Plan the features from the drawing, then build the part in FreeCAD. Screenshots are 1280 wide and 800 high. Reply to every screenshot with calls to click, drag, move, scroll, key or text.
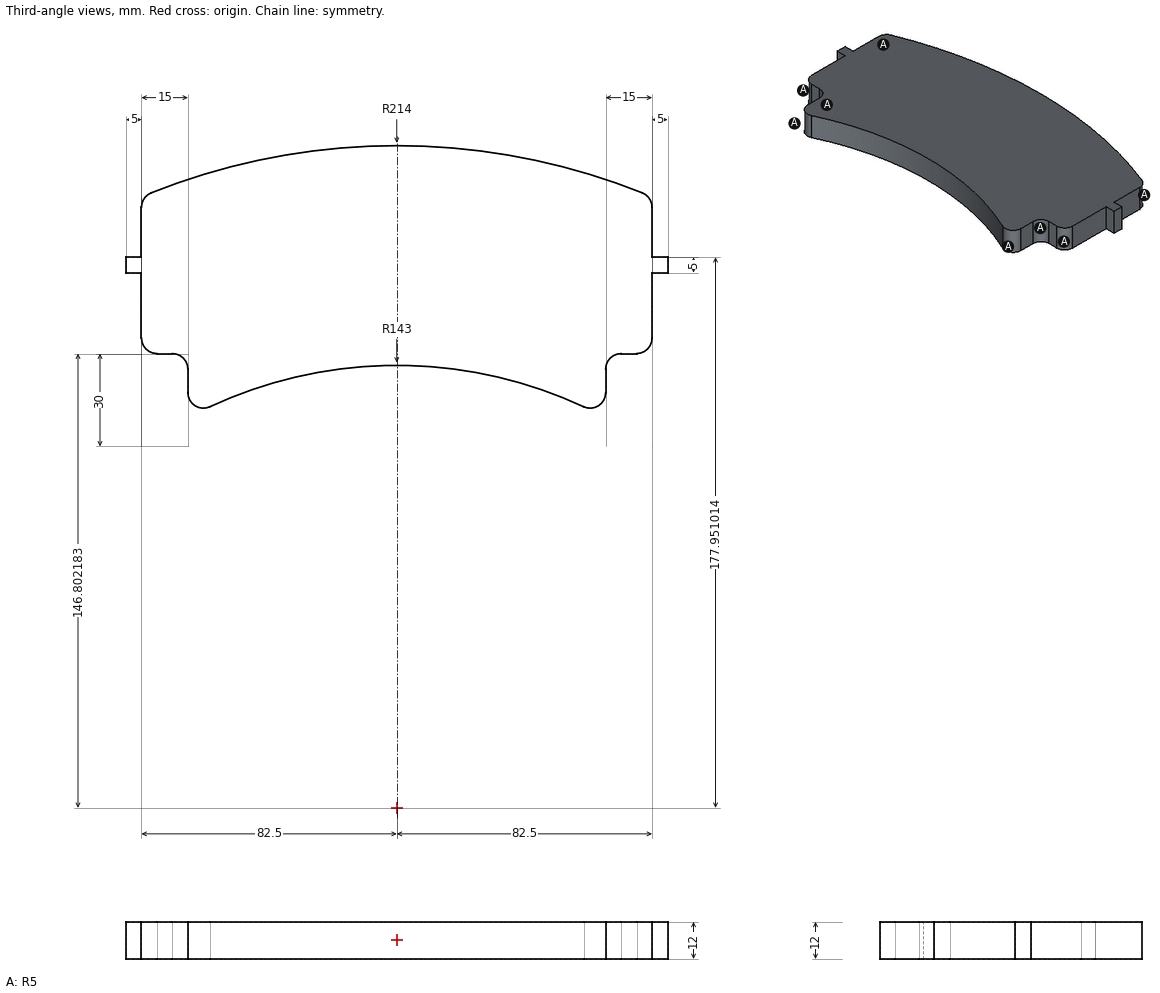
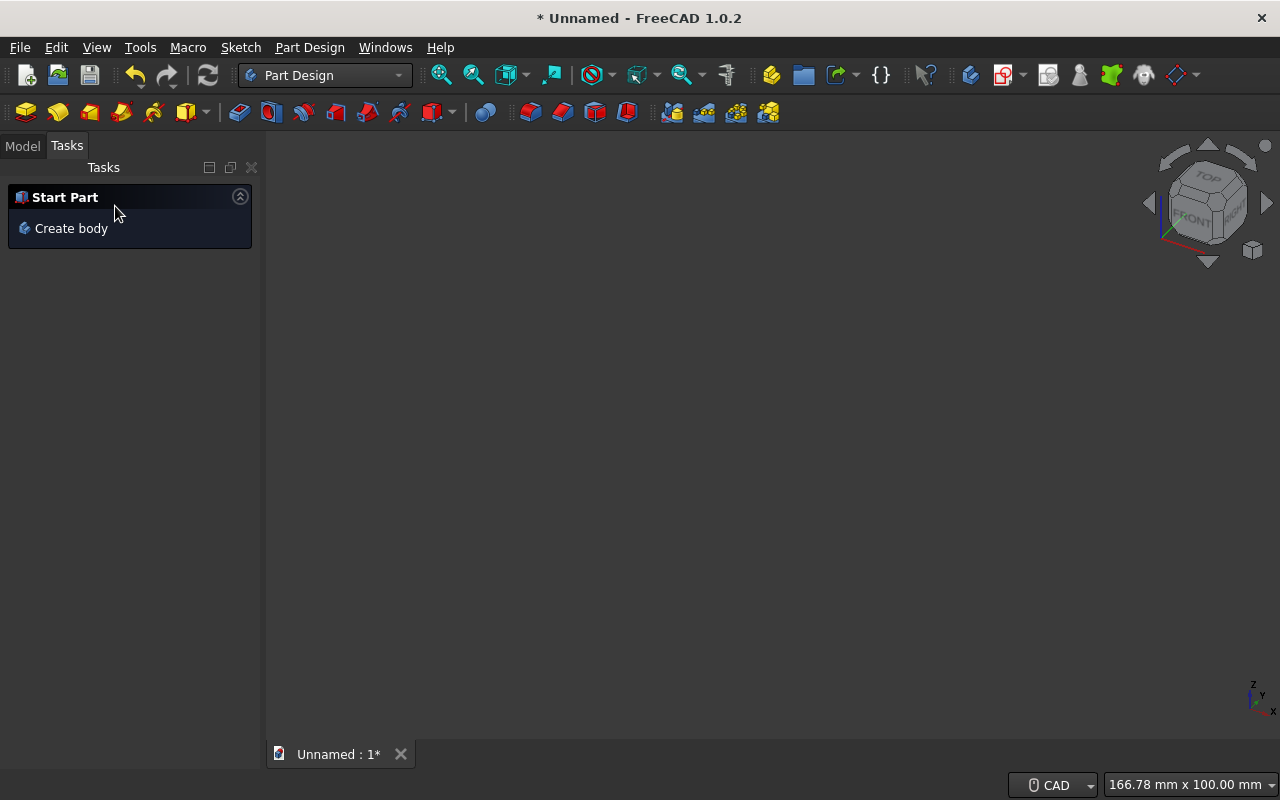
click(442, 76)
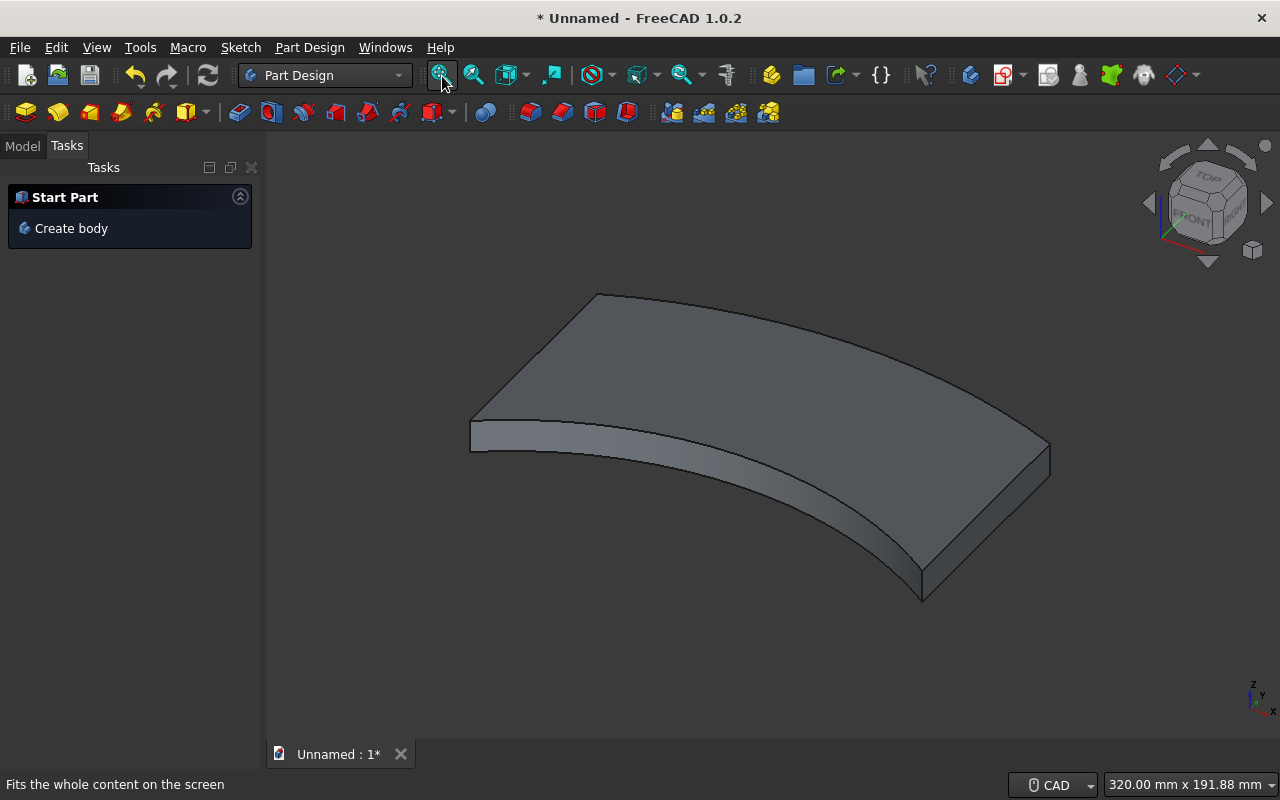
click(795, 397)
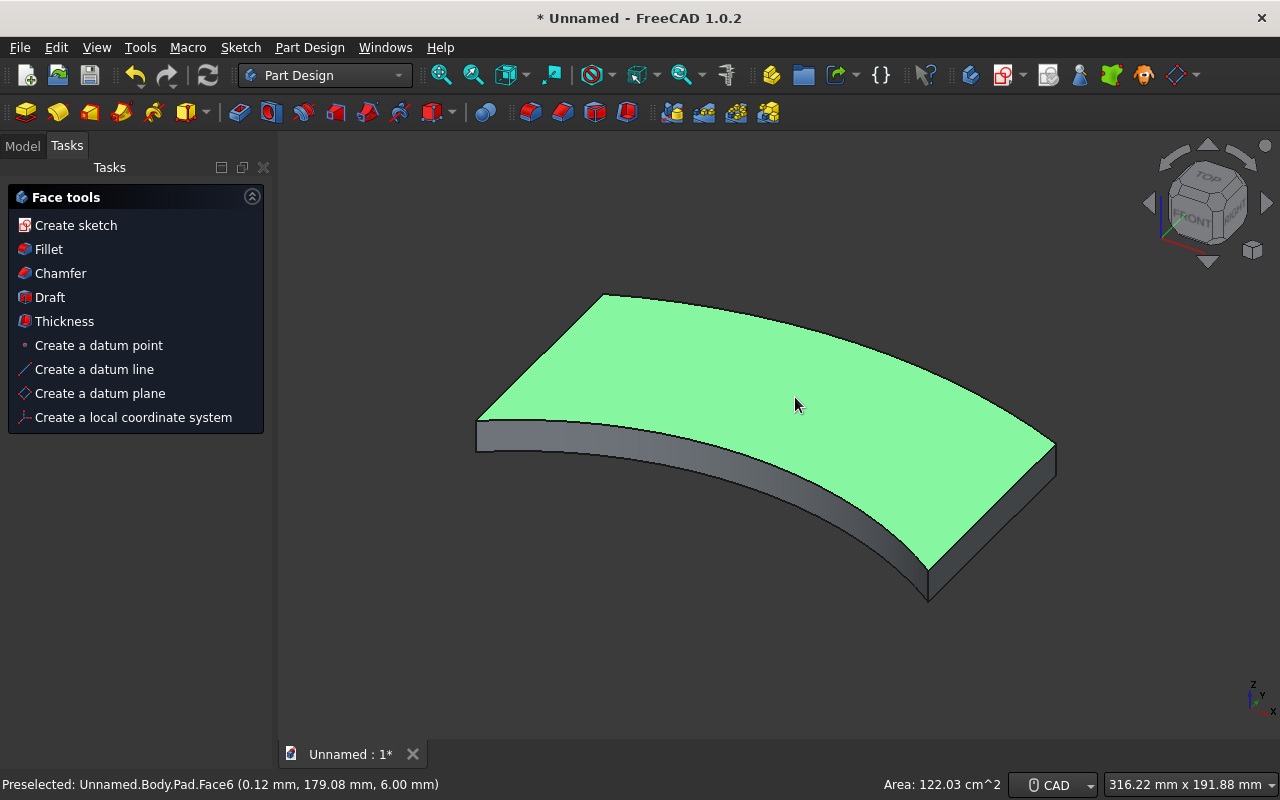
click(1004, 76)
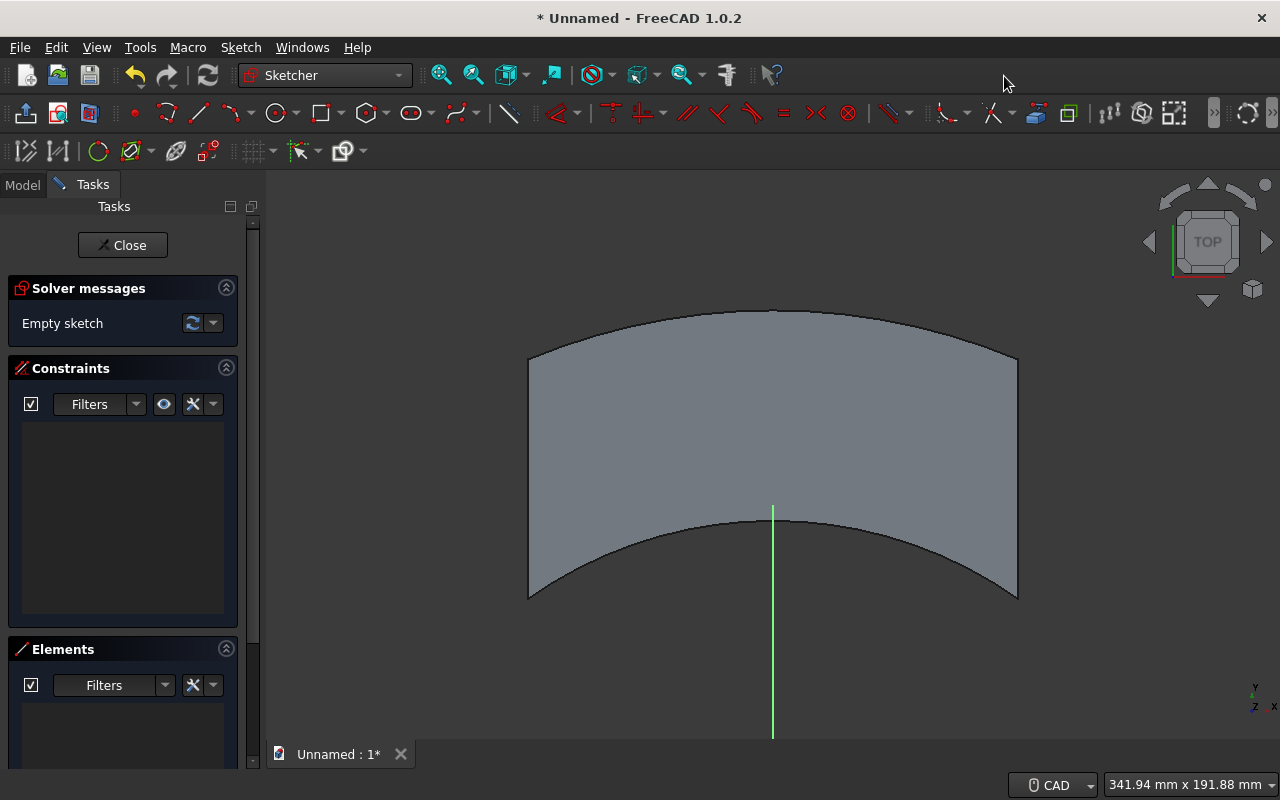
scroll(621, 198, down, 3)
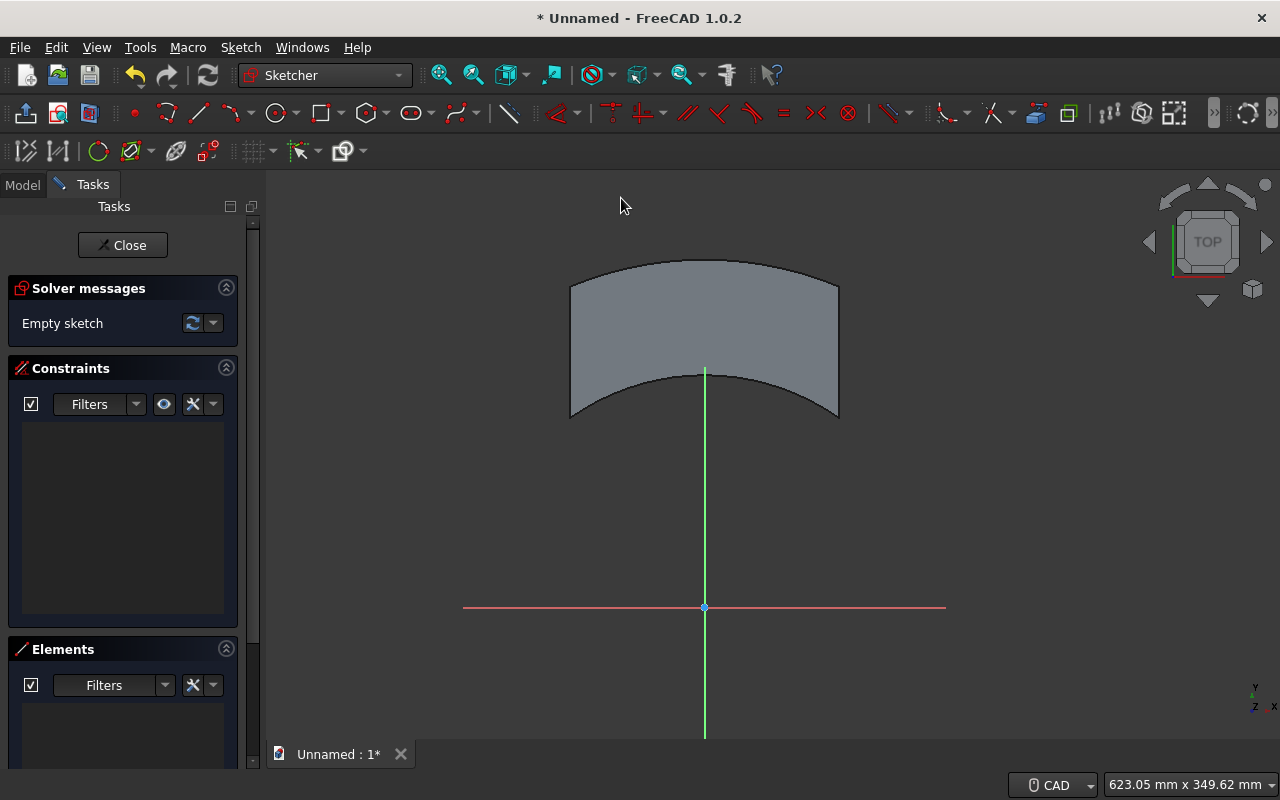
scroll(705, 558, up, 2)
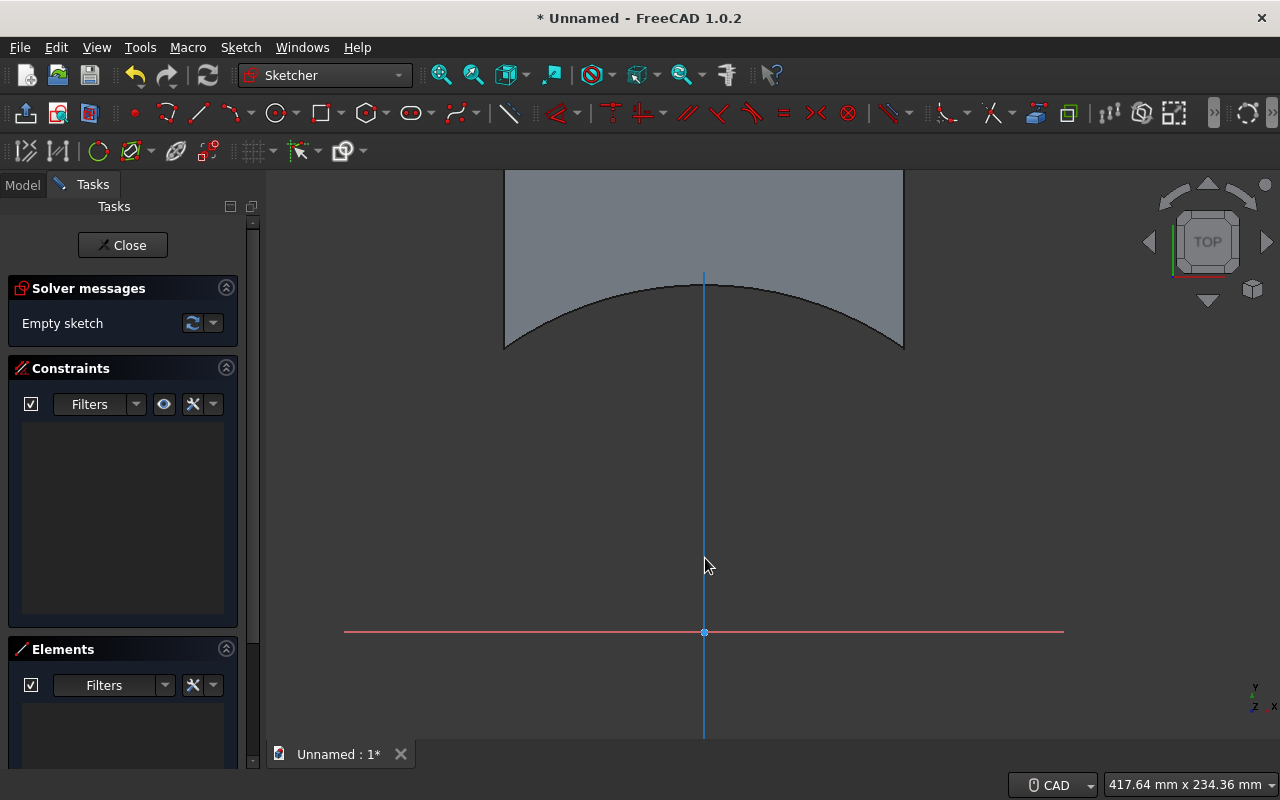
click(322, 114)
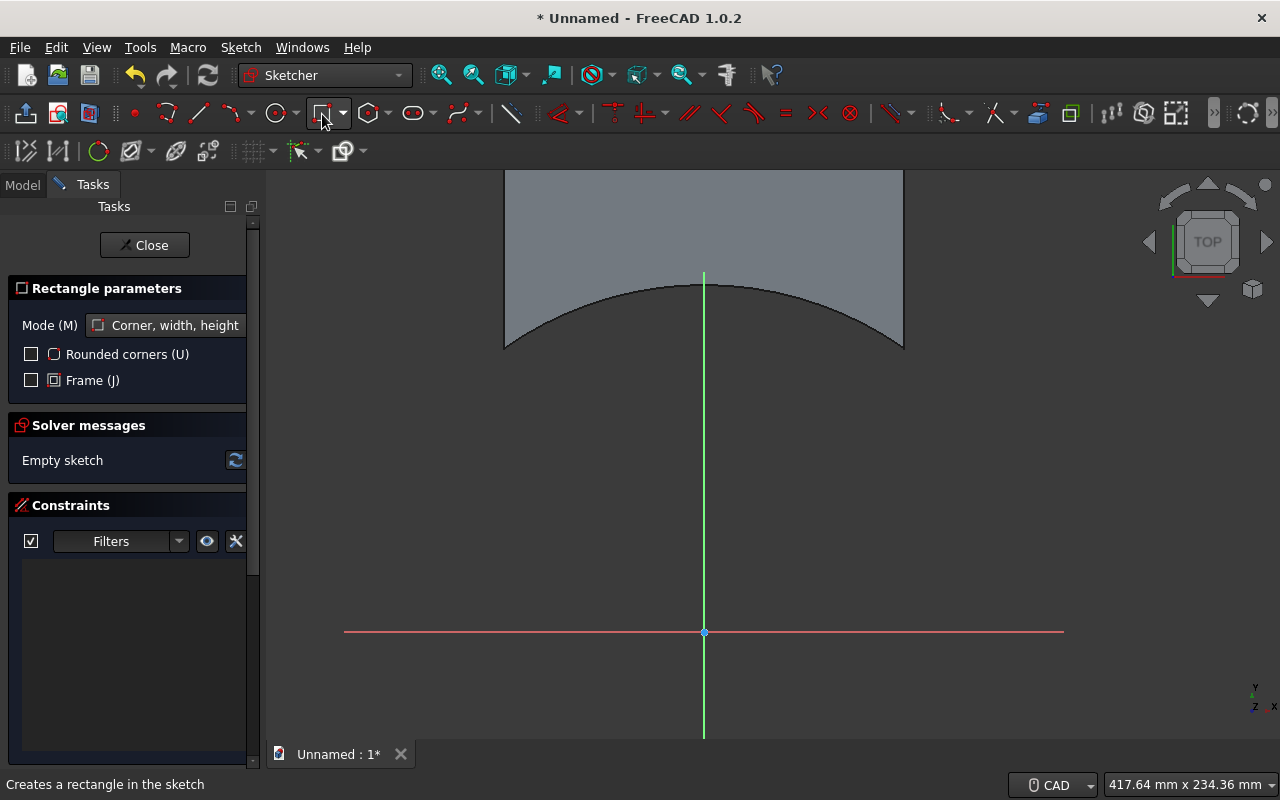
click(504, 276)
move(540, 349)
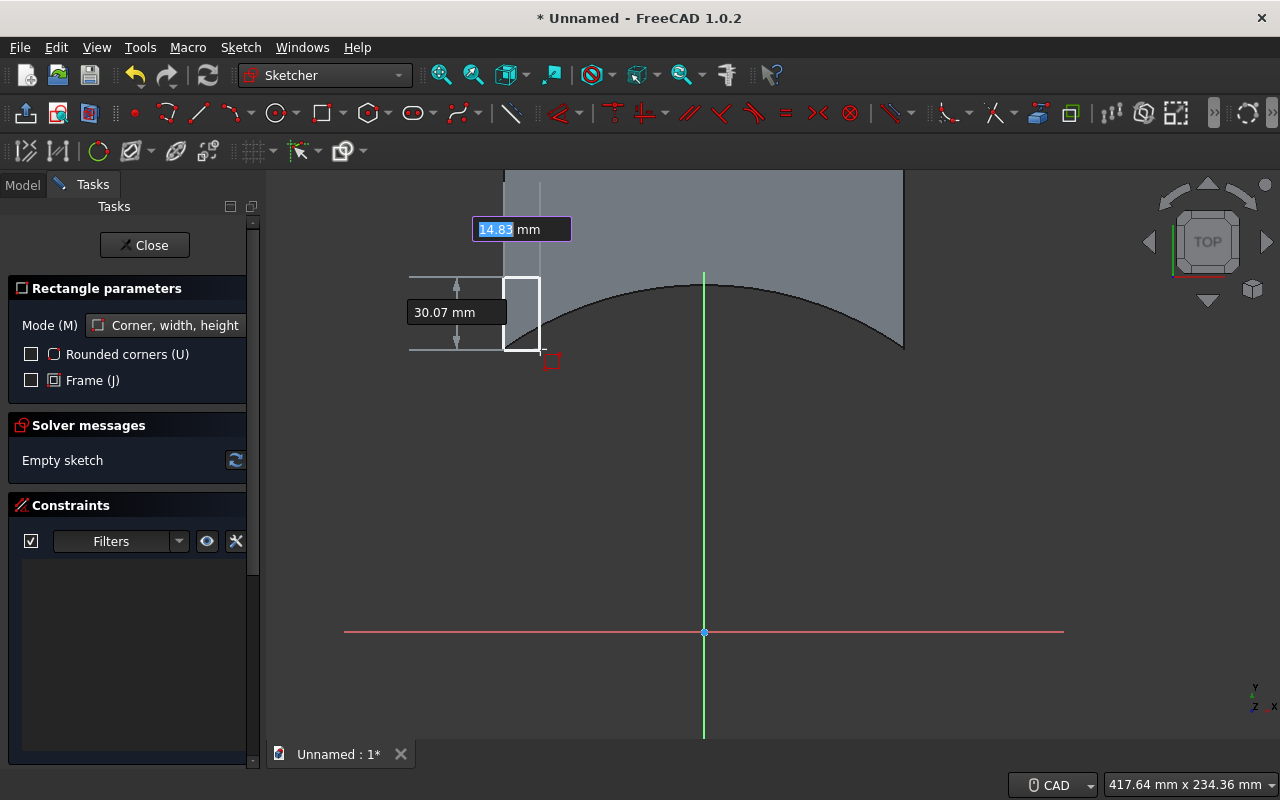
text(15)
key(Tab)
text(30)
key(Return)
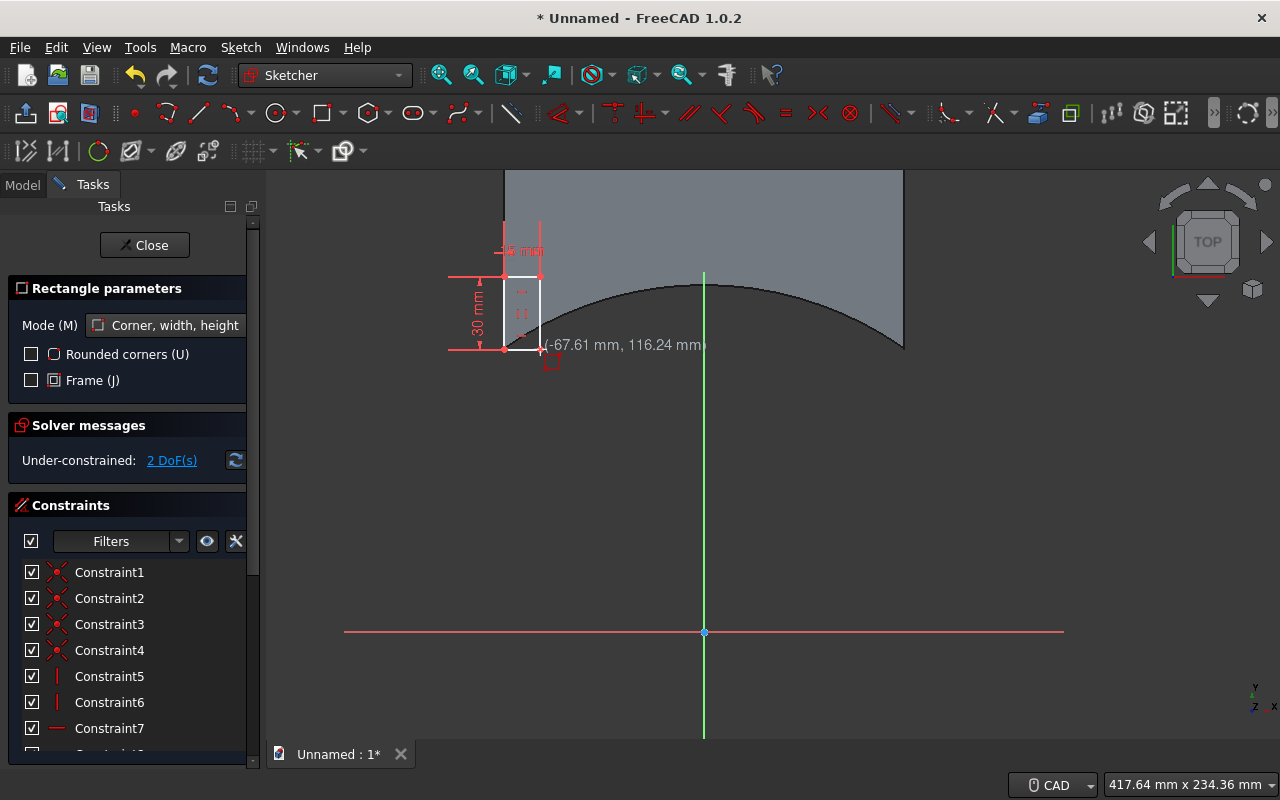
click(868, 276)
move(904, 349)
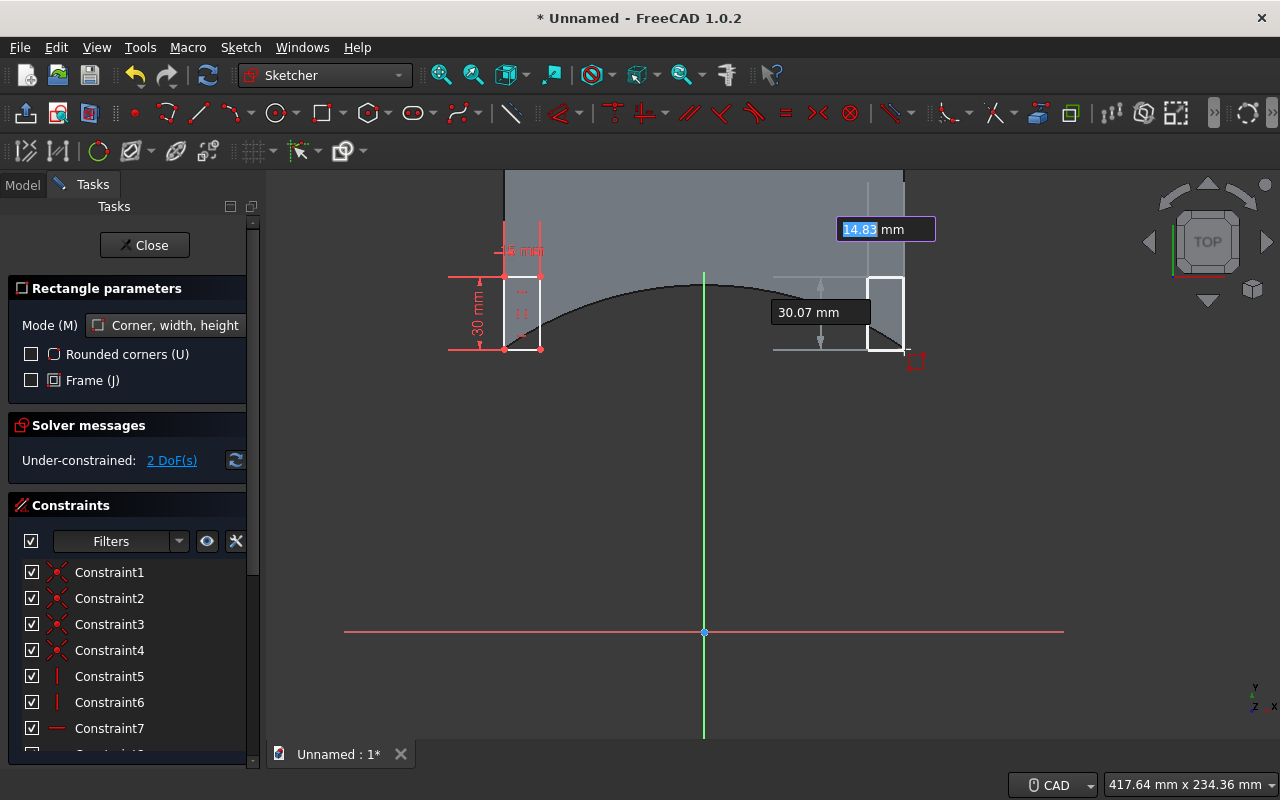
text(15)
key(Tab)
text(30)
key(Return)
key(Escape)